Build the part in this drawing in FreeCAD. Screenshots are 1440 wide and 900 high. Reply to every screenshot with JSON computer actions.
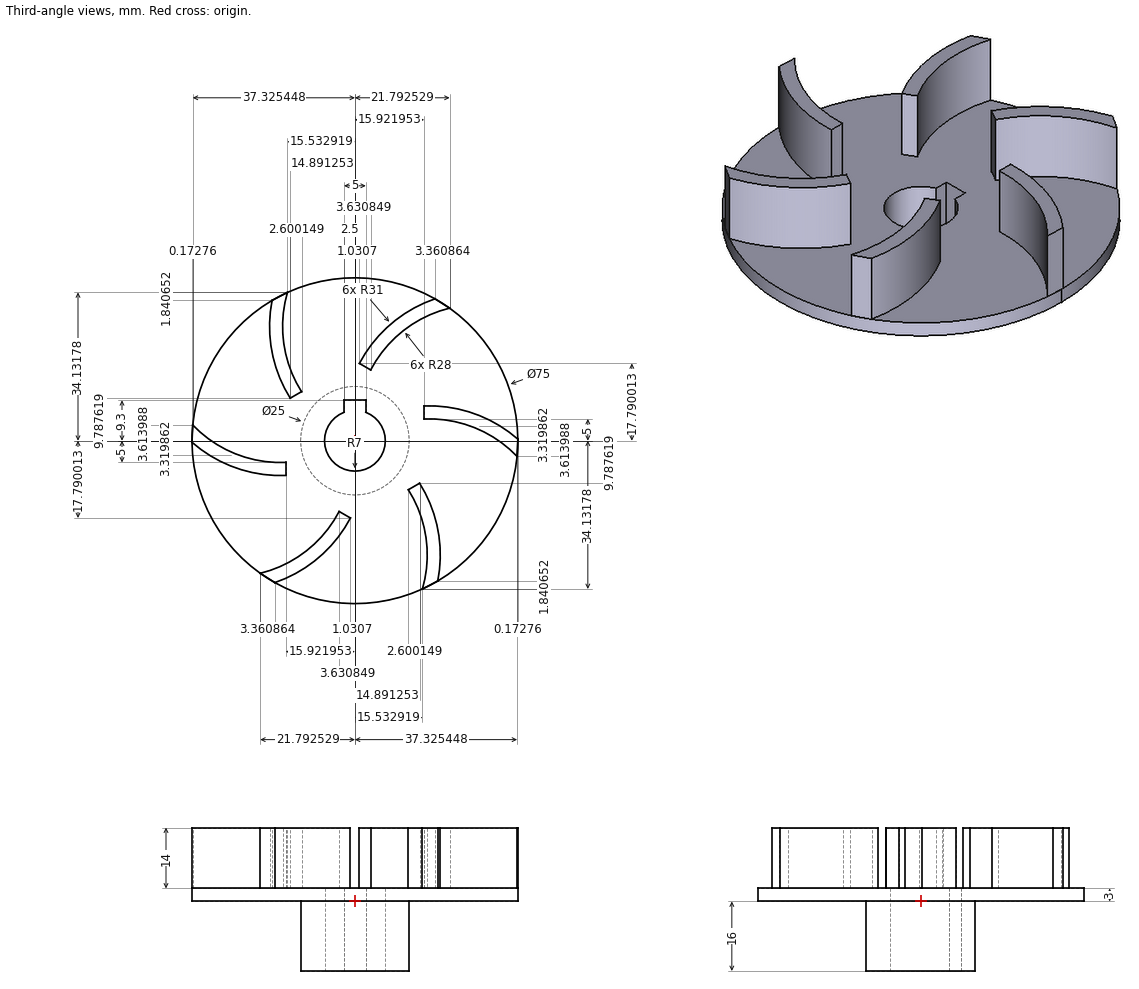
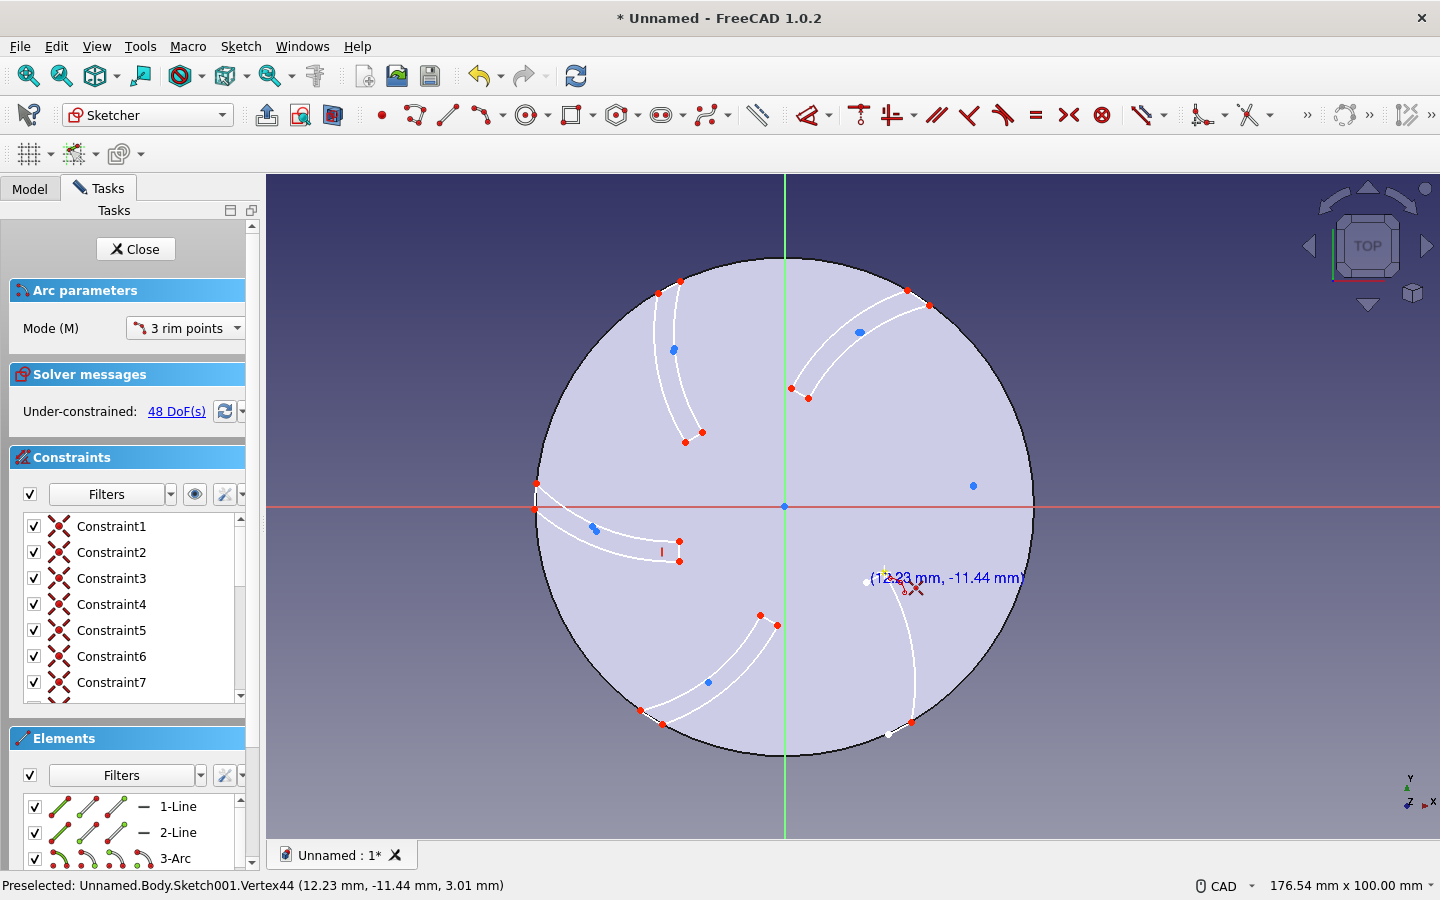
{"action": "left_click", "coordinate": [888, 735]}
{"action": "left_click", "coordinate": [894, 656]}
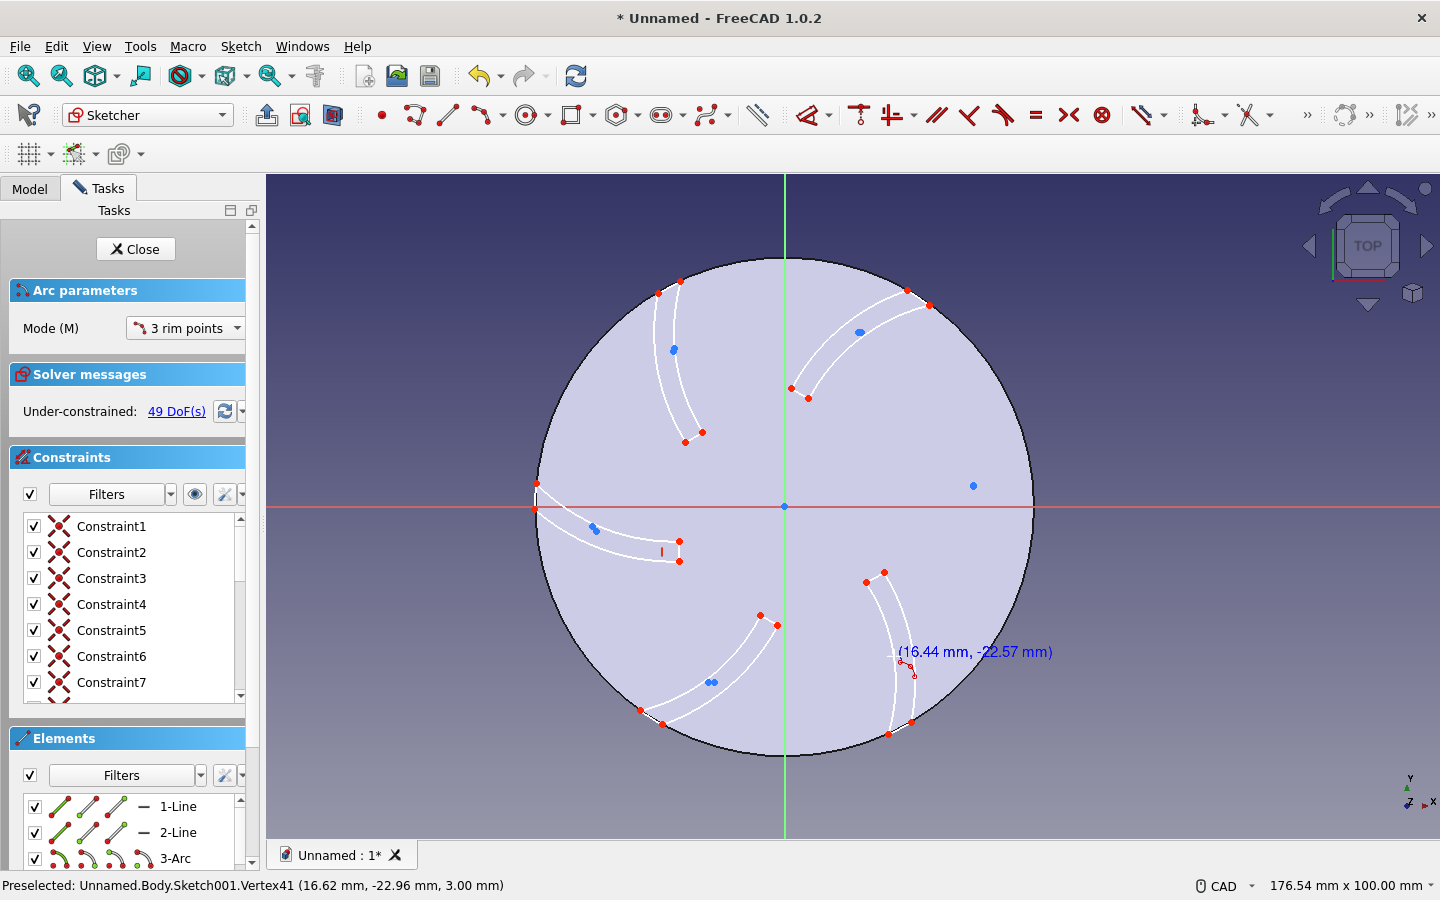
{"action": "left_click", "coordinate": [448, 116]}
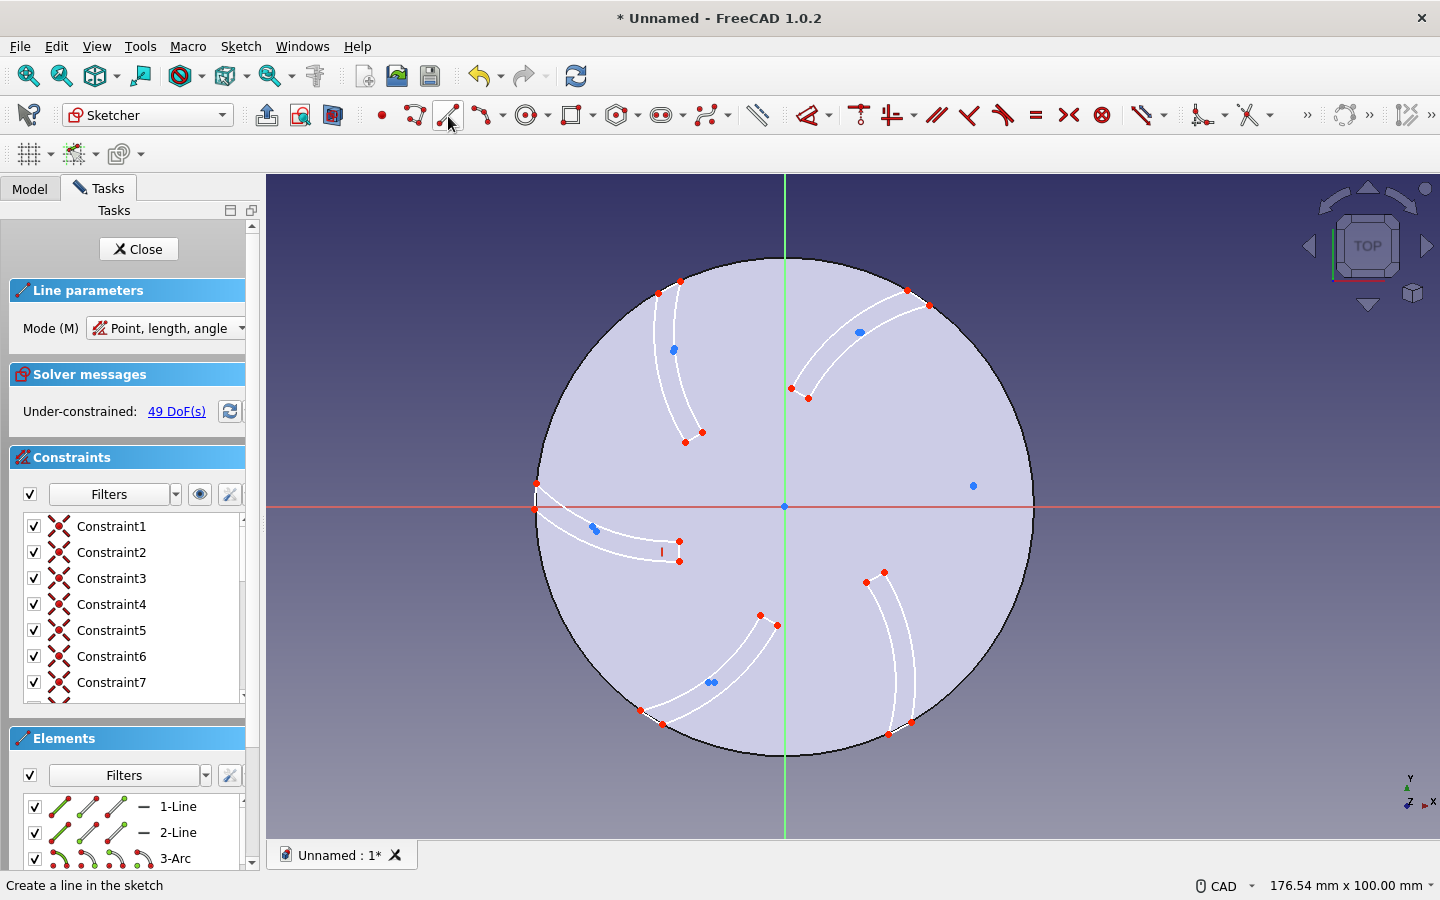
{"action": "left_click", "coordinate": [1033, 531]}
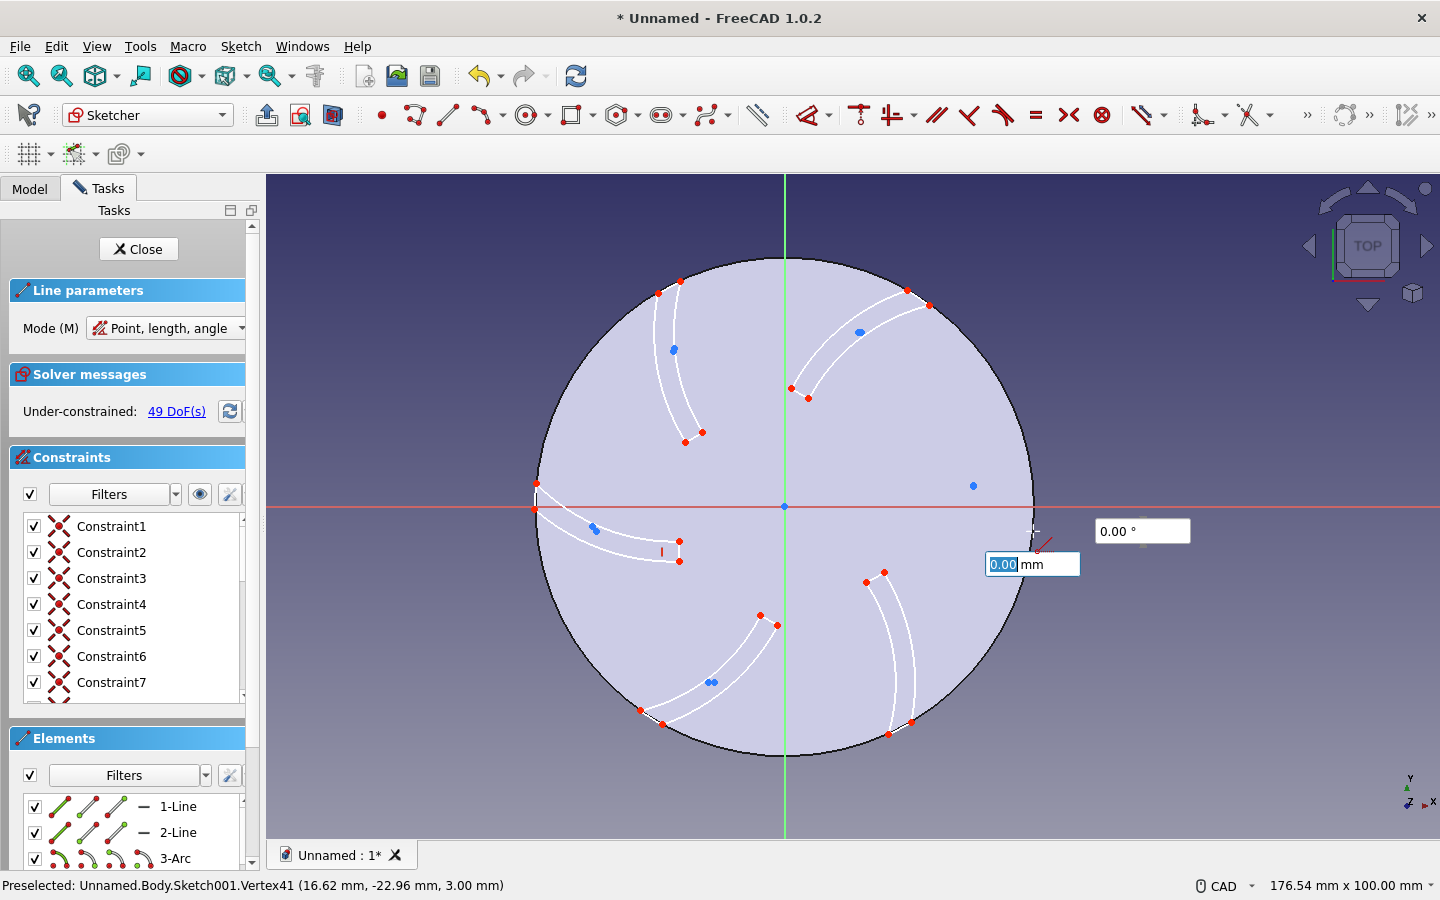
{"action": "scroll", "coordinate": [1034, 504], "scroll_direction": "up", "scroll_amount": 10}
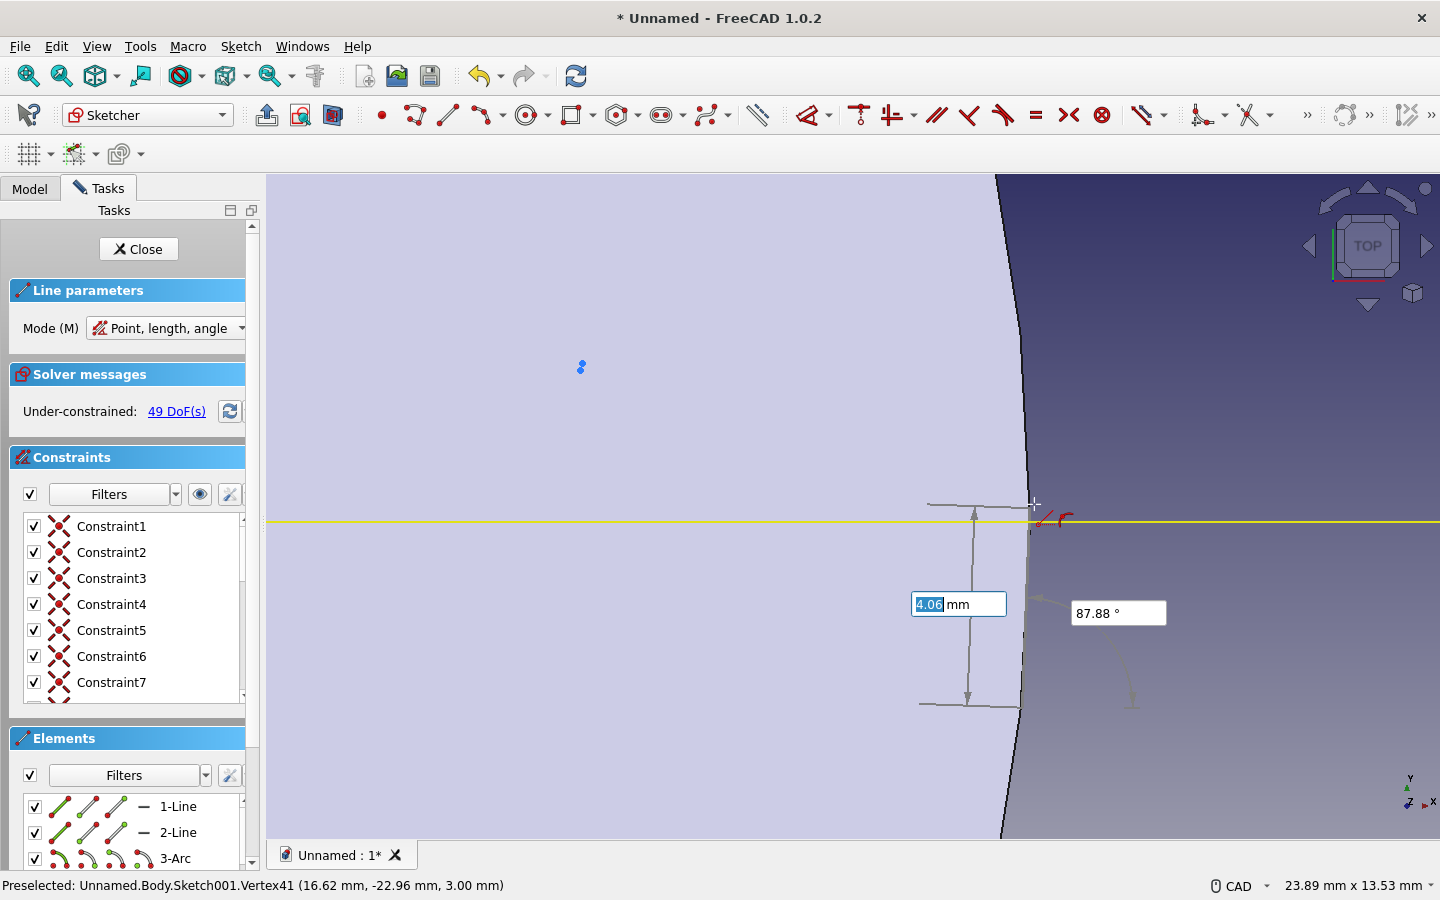
{"action": "left_click", "coordinate": [1033, 504]}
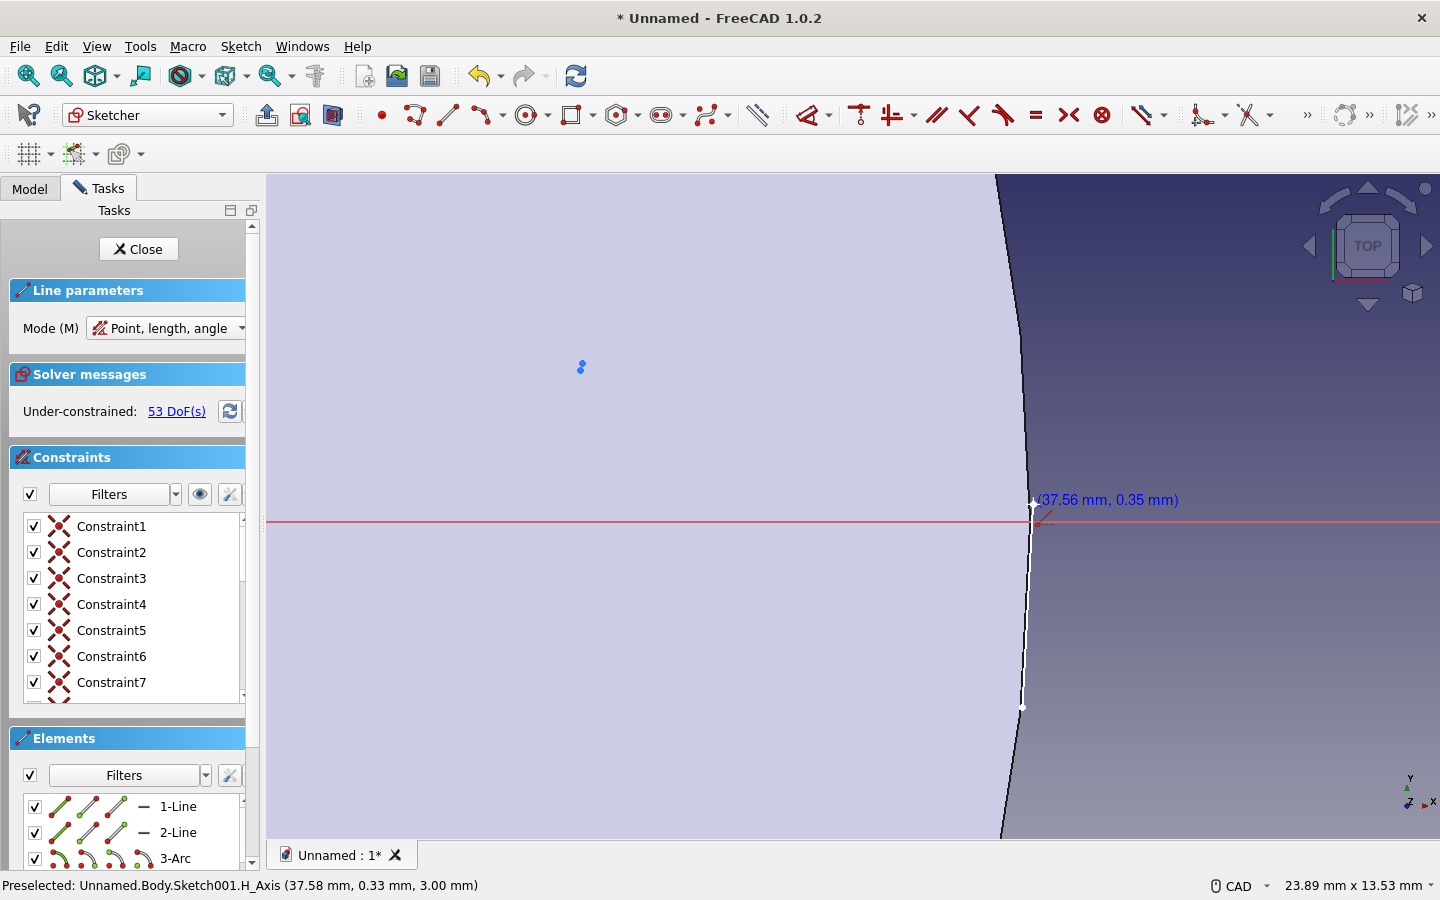
{"action": "scroll", "coordinate": [1034, 504], "scroll_direction": "down", "scroll_amount": 10}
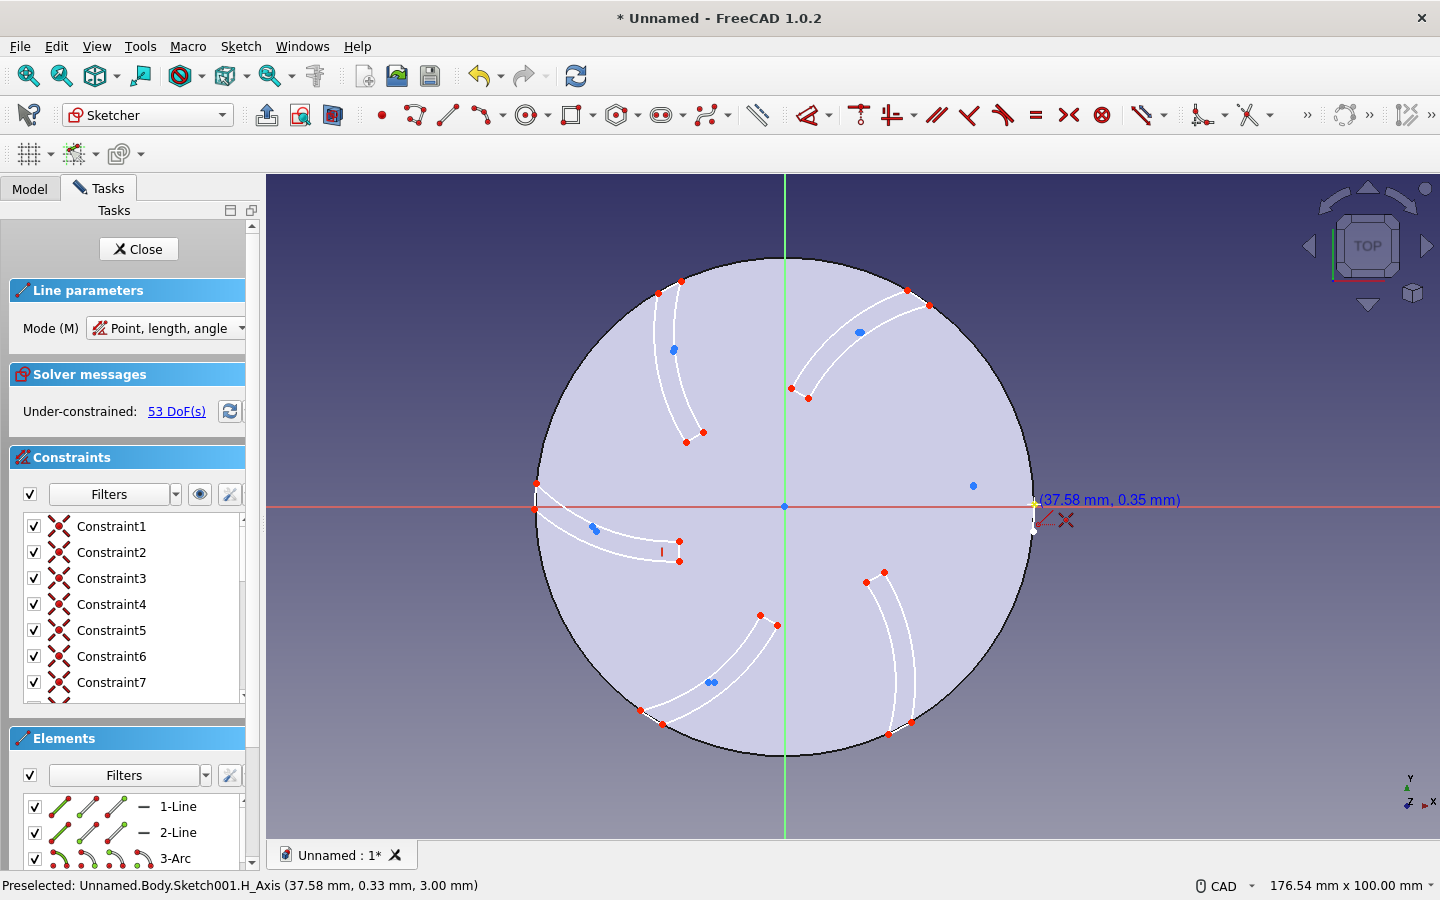
{"action": "left_click", "coordinate": [891, 454]}
{"action": "left_click", "coordinate": [891, 474]}